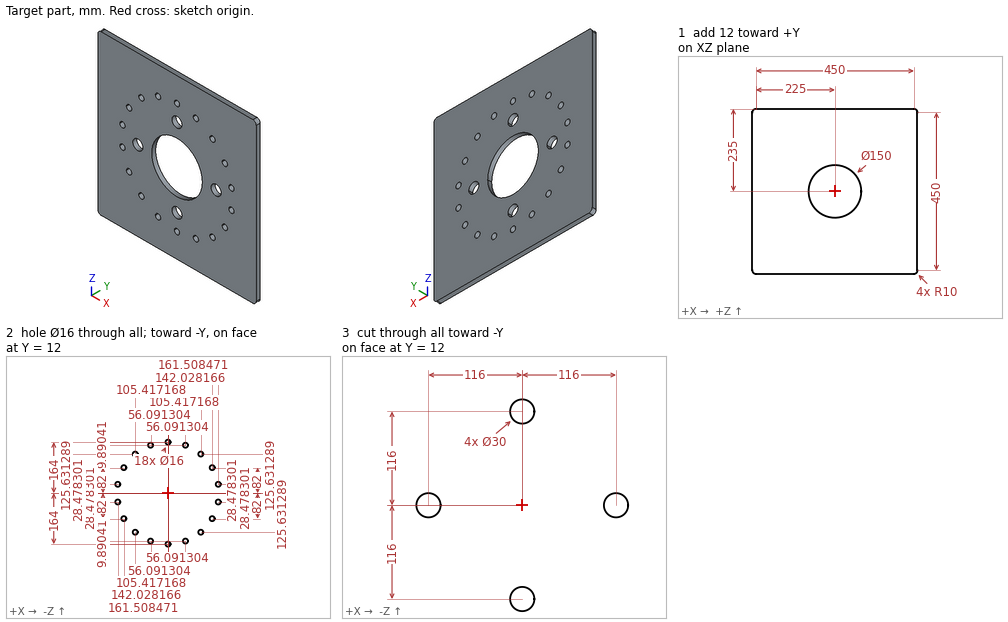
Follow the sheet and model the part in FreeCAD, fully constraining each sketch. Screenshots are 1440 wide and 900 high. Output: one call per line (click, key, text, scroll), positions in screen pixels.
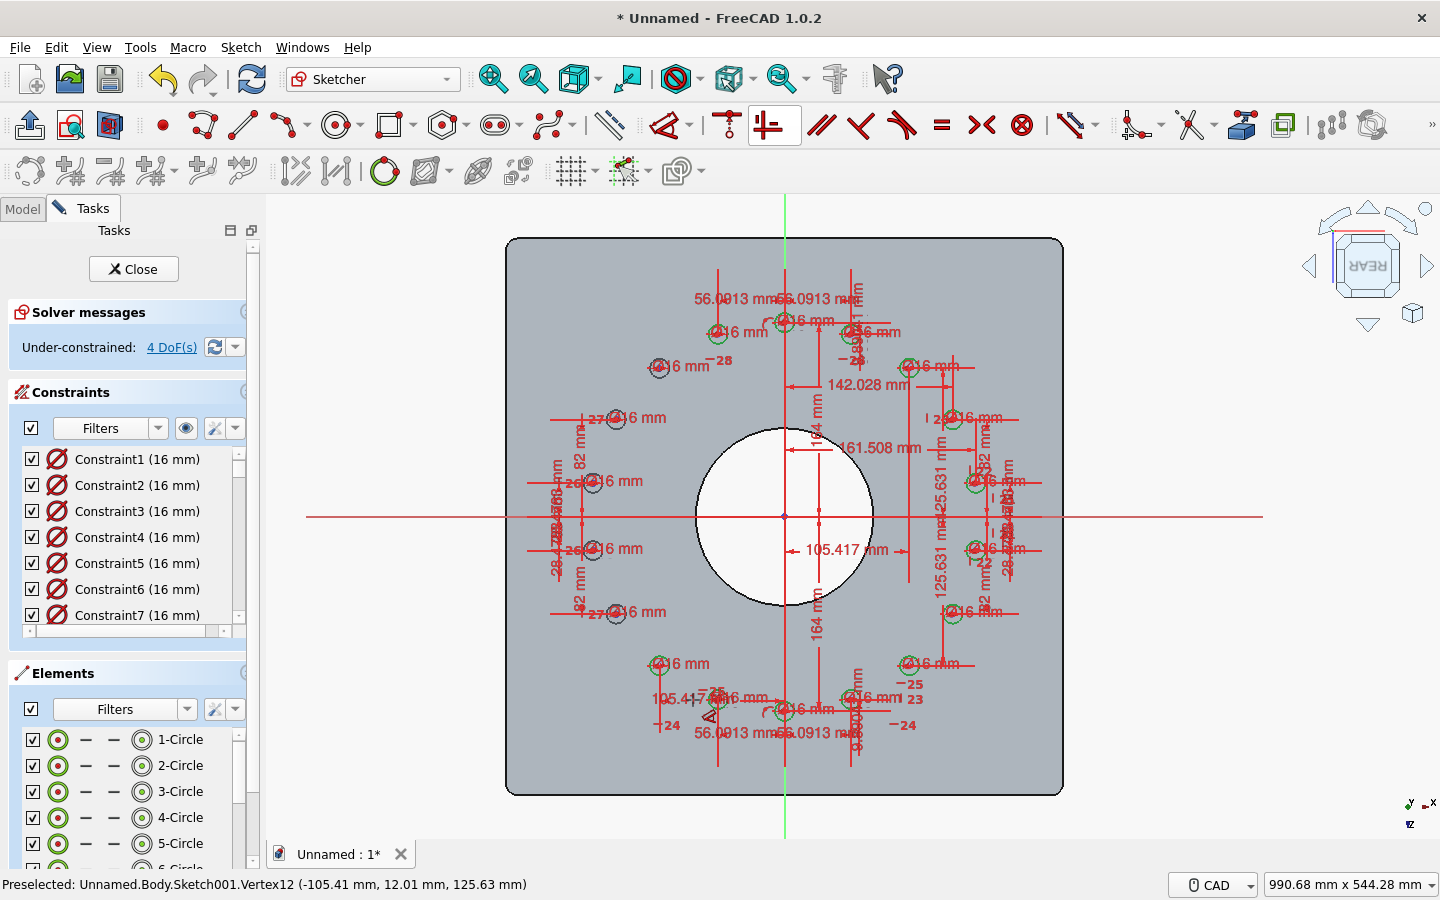
click(616, 614)
click(700, 648)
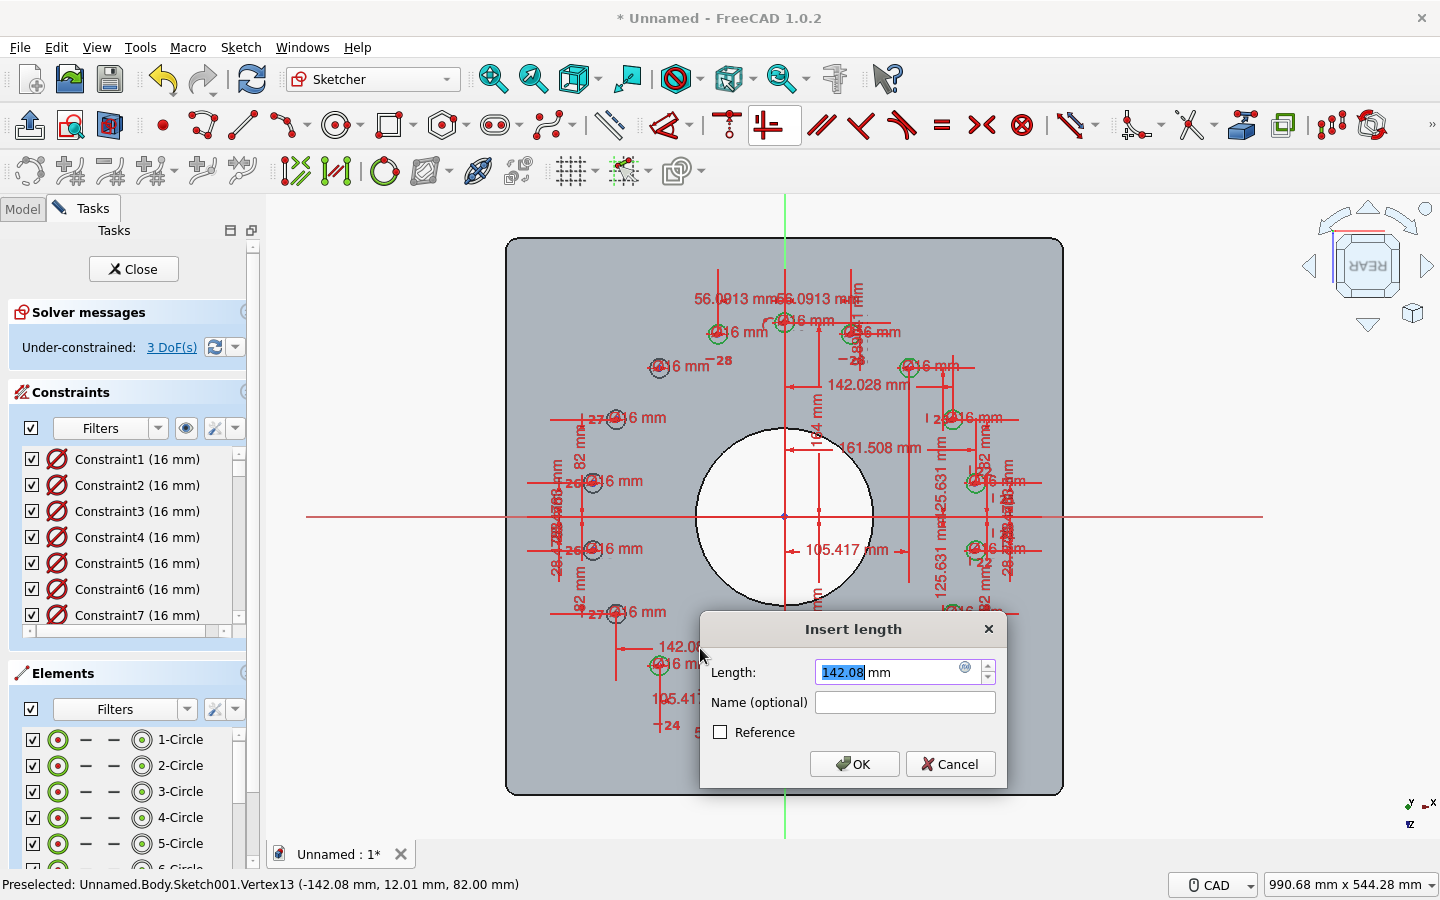
text(142.028166)
key(Return)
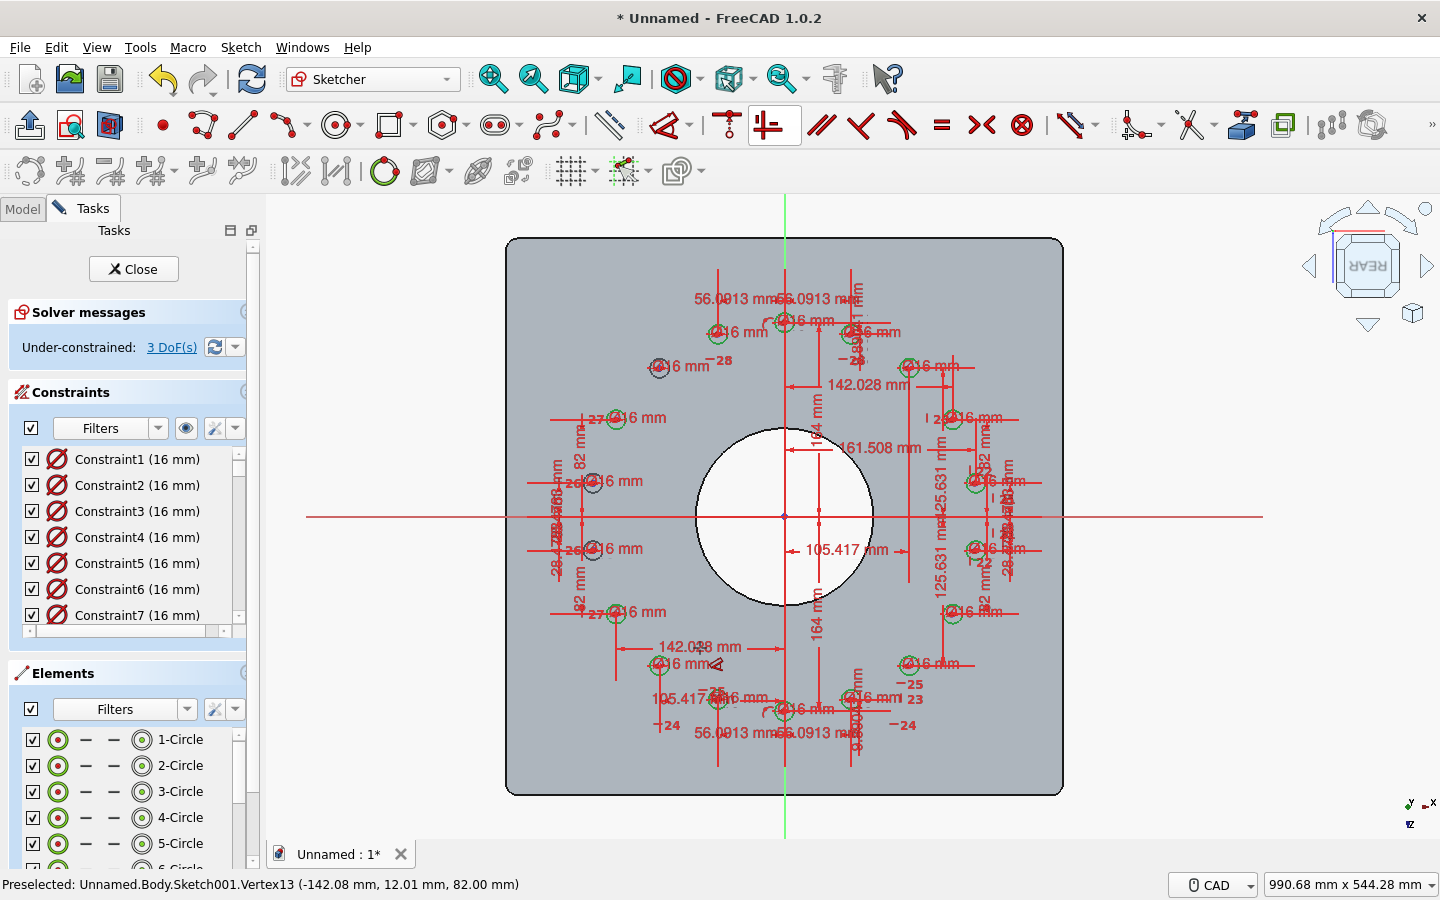
click(593, 551)
click(689, 585)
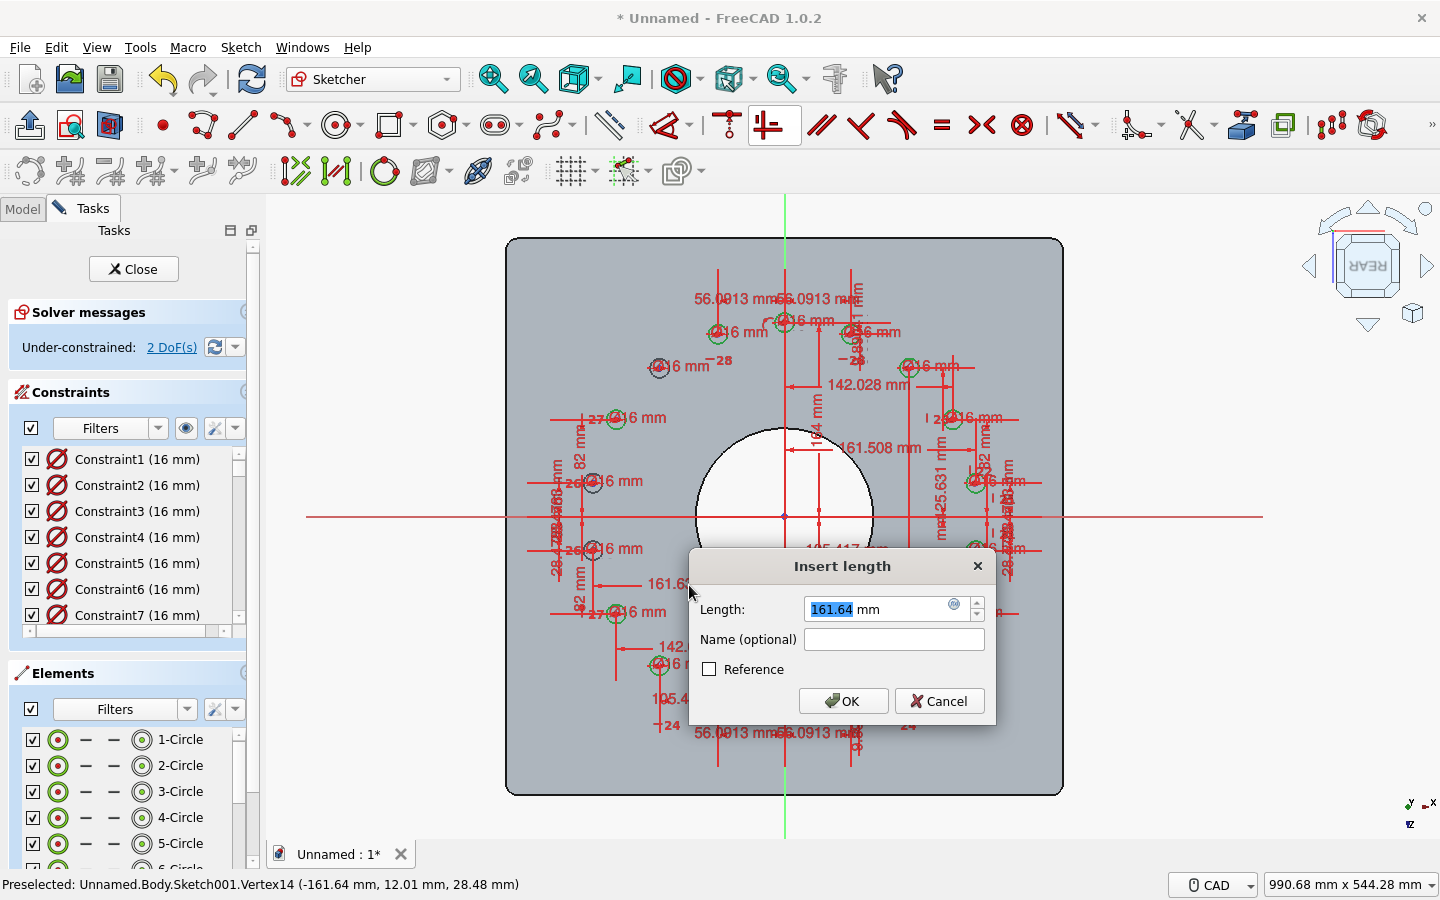
text(161.508471)
key(Return)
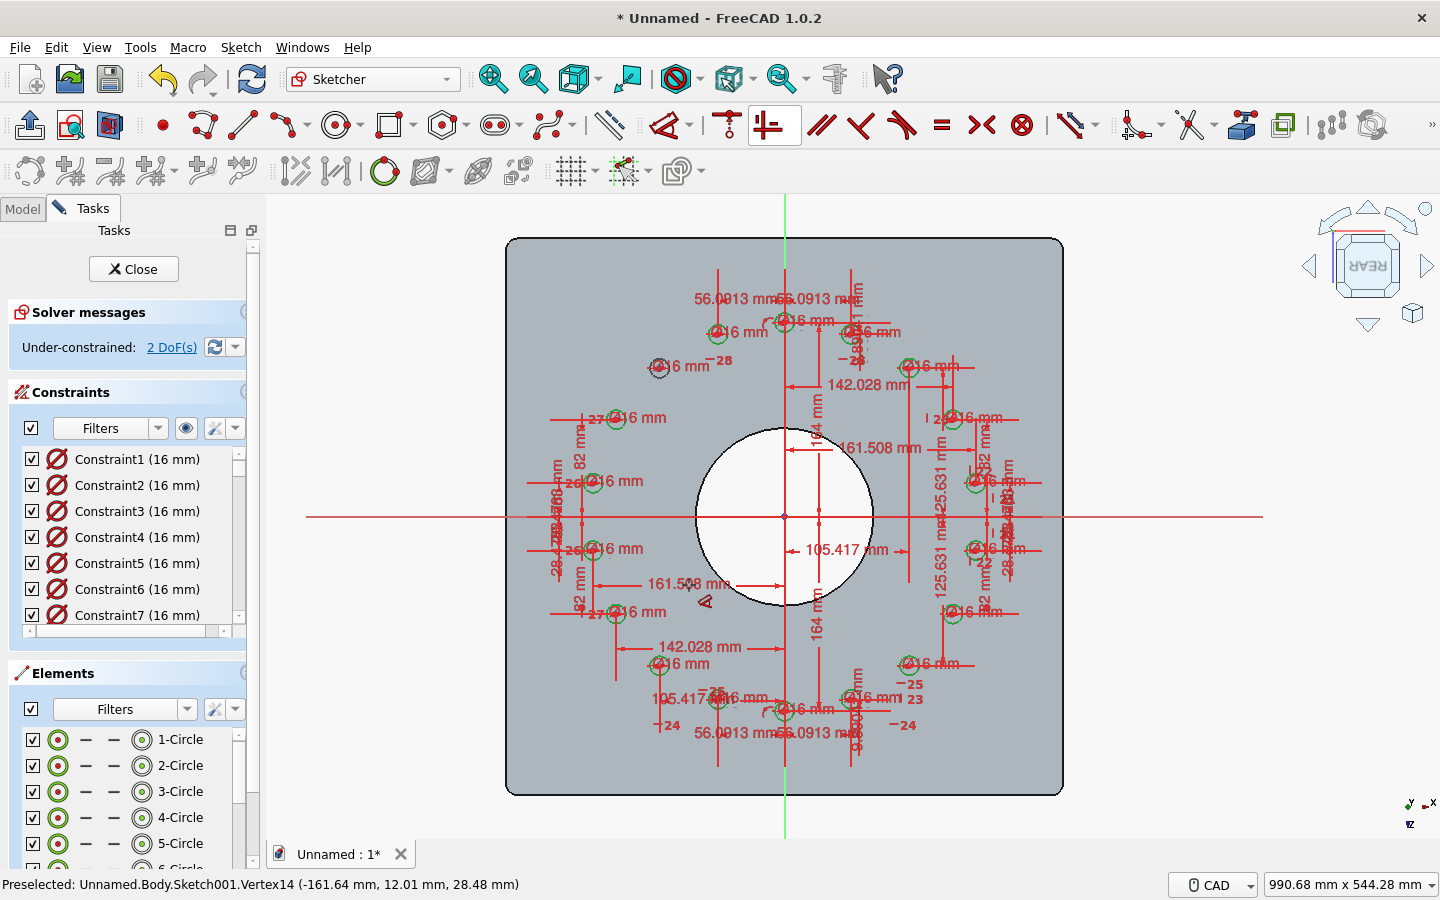
click(660, 368)
click(693, 334)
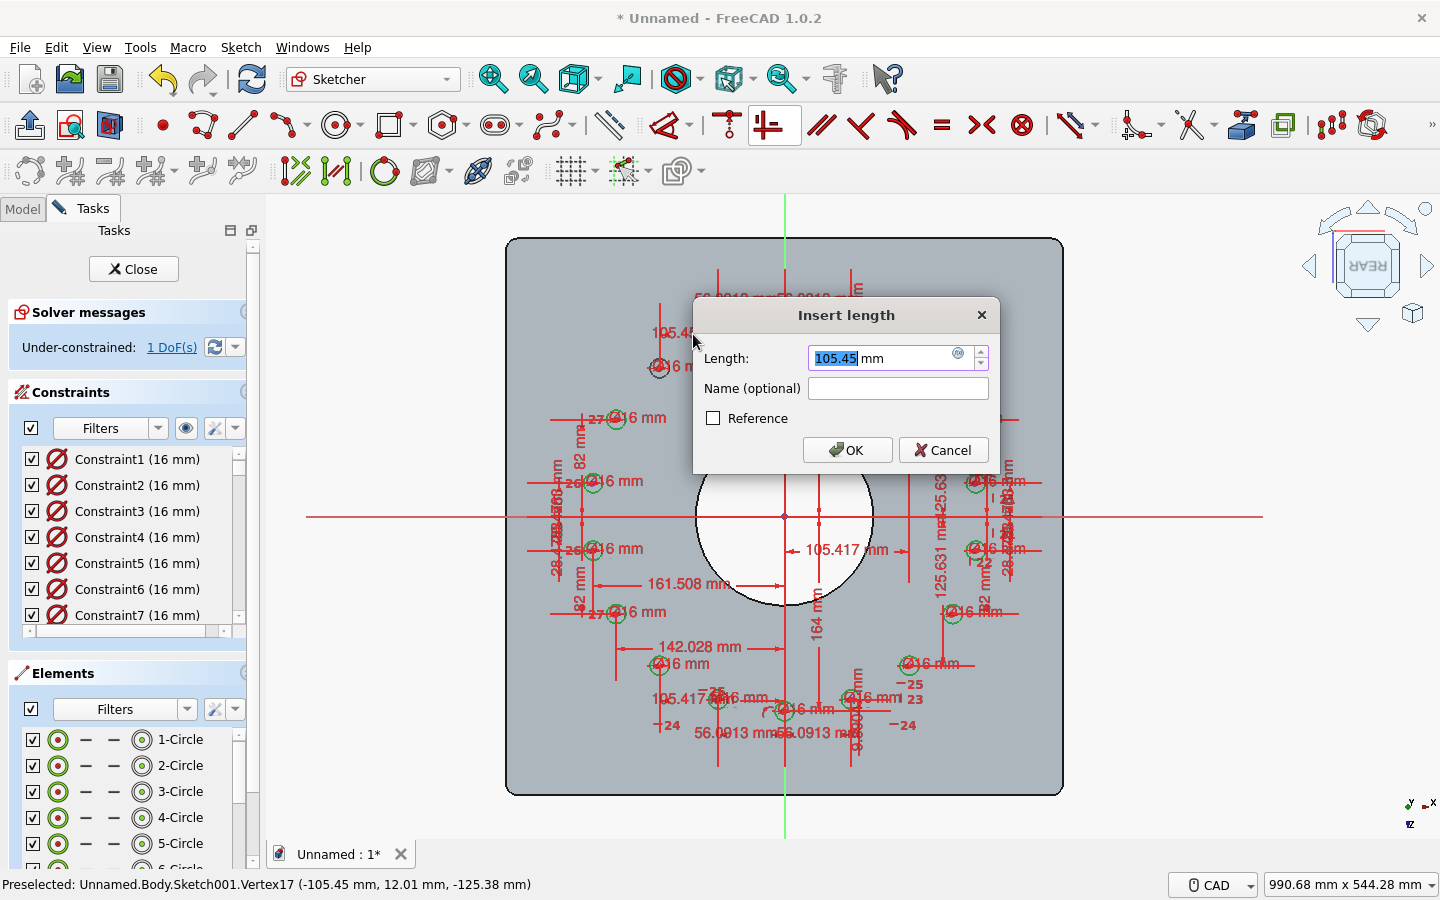
text(105.417168)
key(Return)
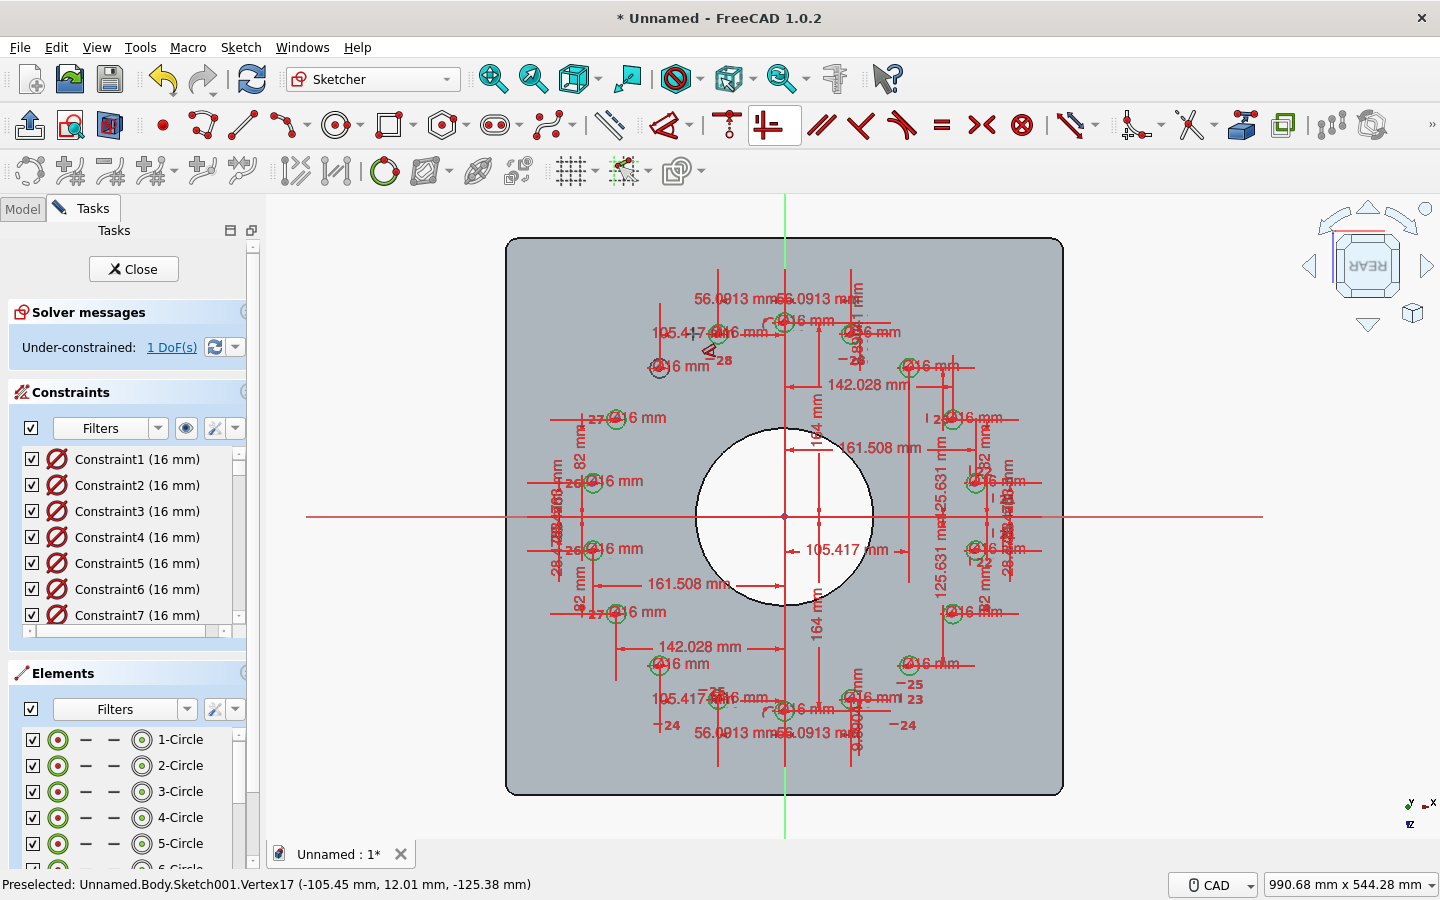
click(660, 368)
click(626, 477)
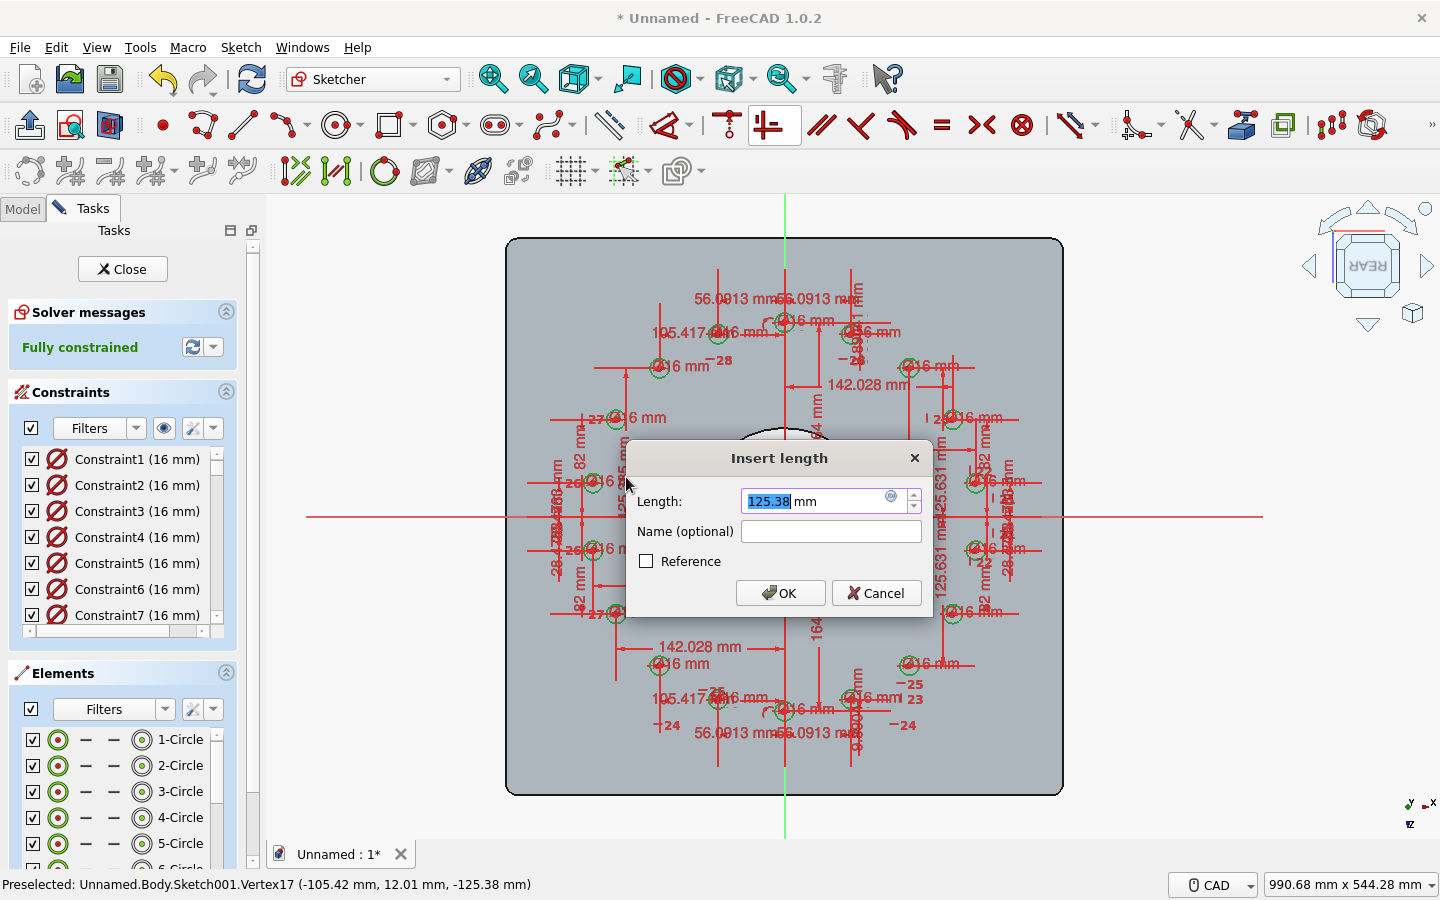
text(125.631289)
key(Return)
key(Escape)